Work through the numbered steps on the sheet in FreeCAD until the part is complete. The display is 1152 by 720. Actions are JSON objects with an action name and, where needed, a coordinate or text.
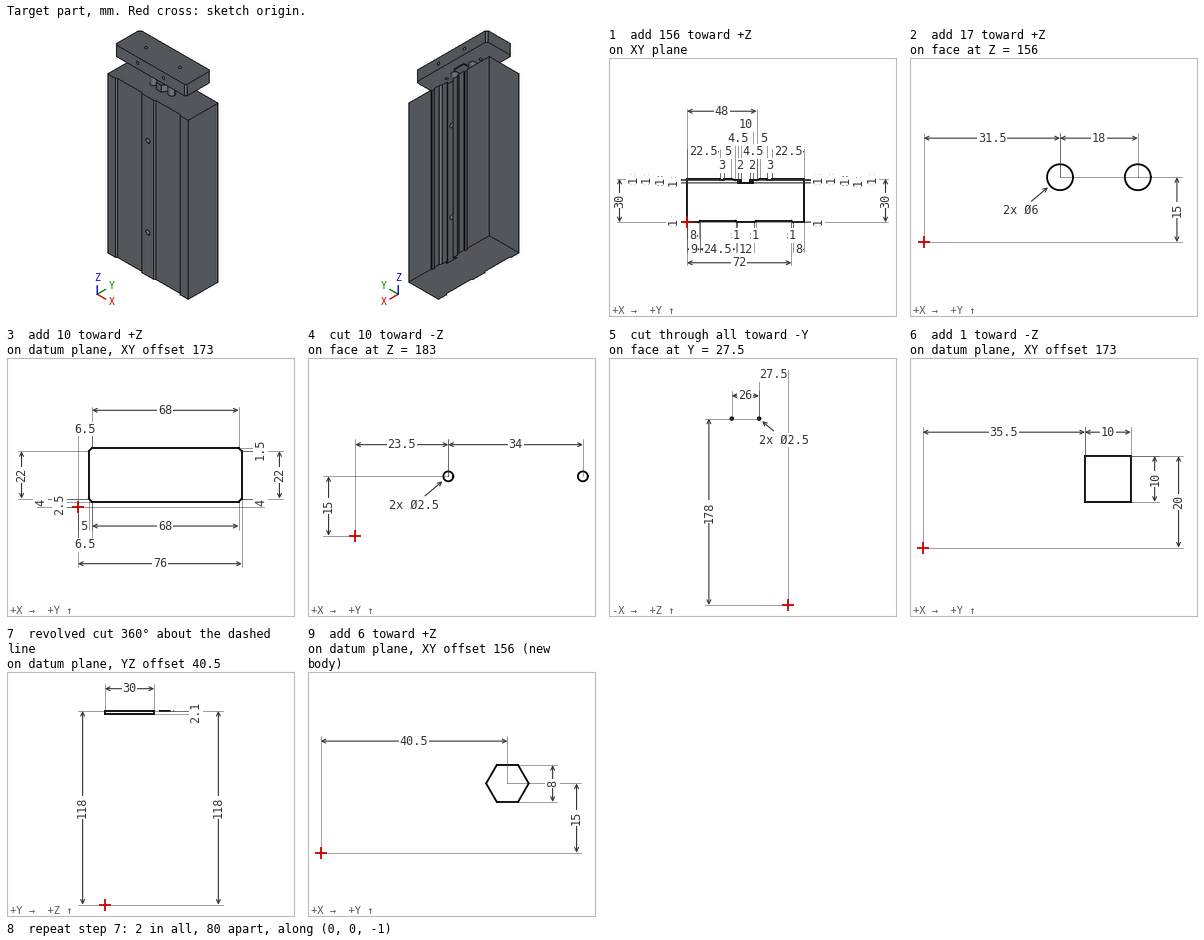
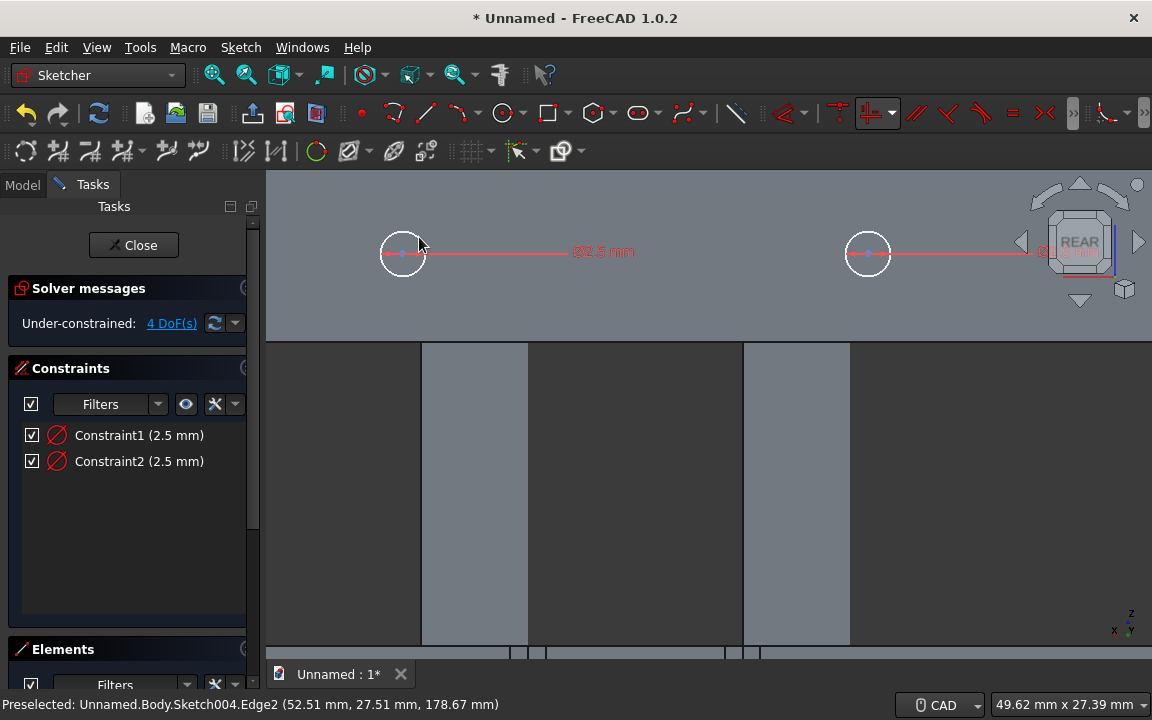
{"action": "left_click", "coordinate": [868, 254]}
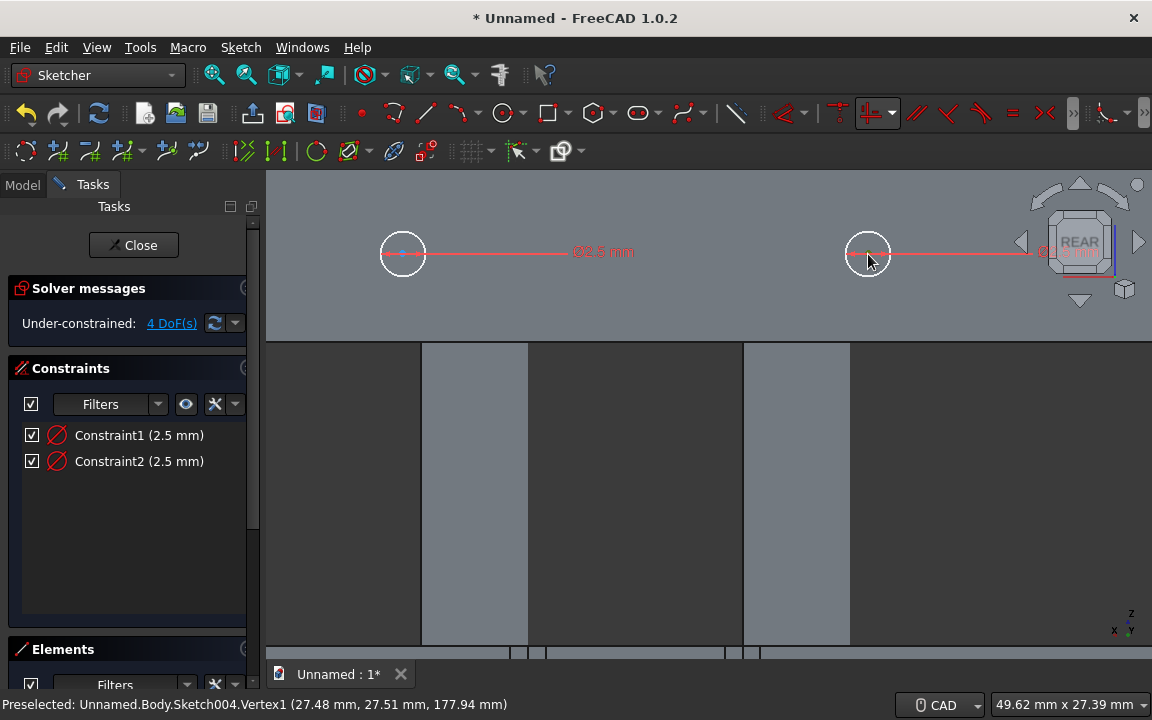
{"action": "left_click", "coordinate": [403, 254]}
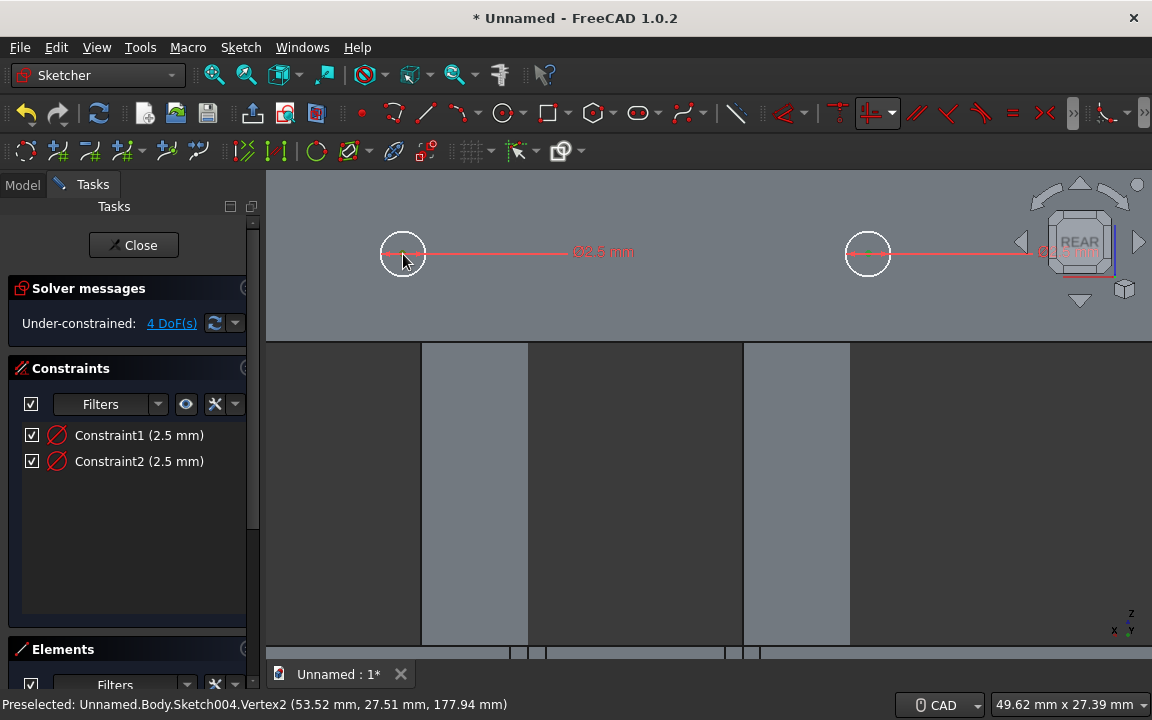
{"action": "key", "text": "h"}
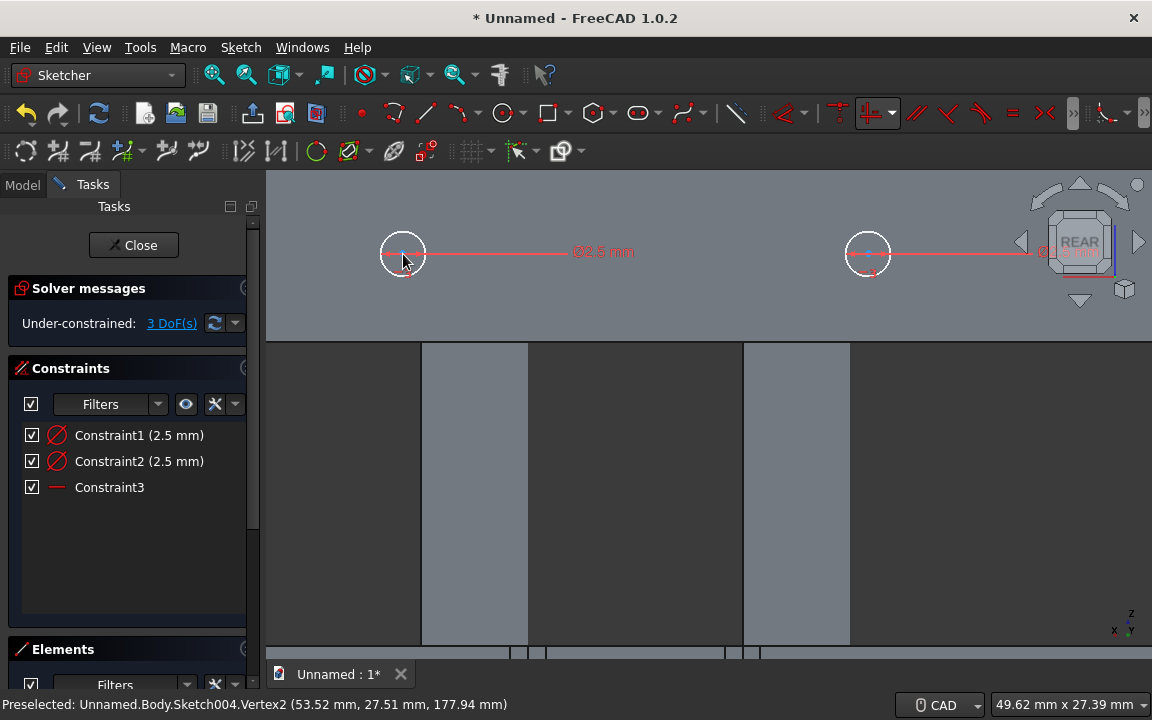
{"action": "key", "text": "d"}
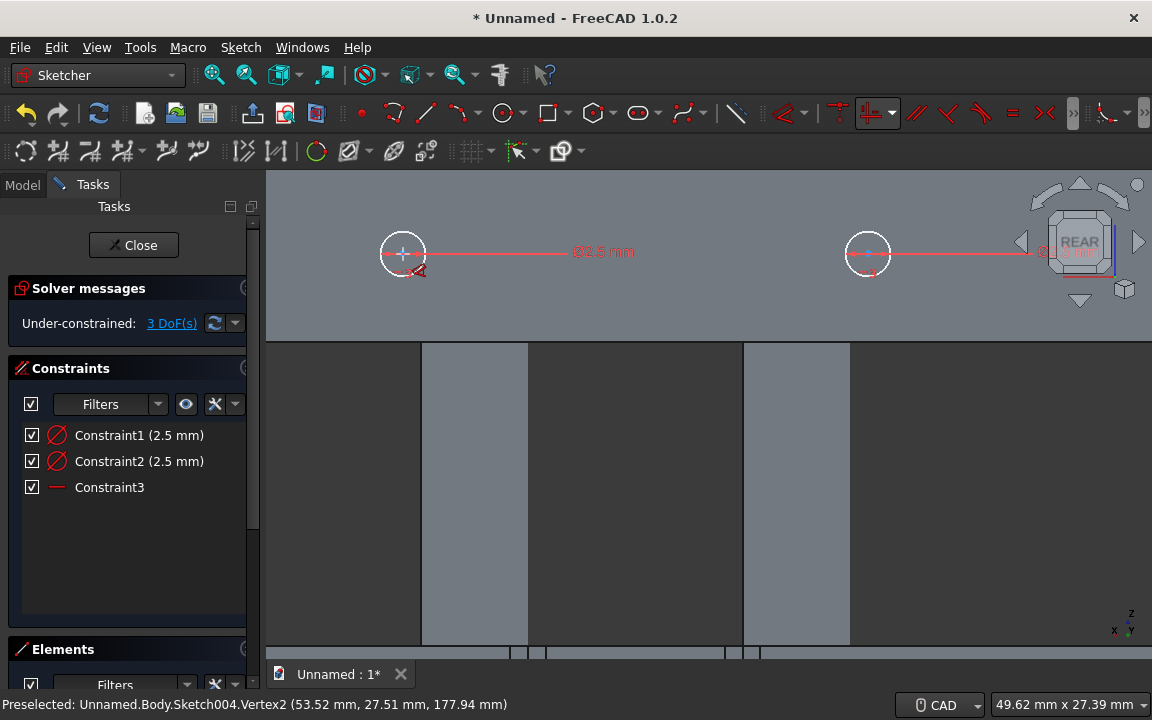
{"action": "left_click", "coordinate": [868, 254]}
{"action": "left_click", "coordinate": [834, 443]}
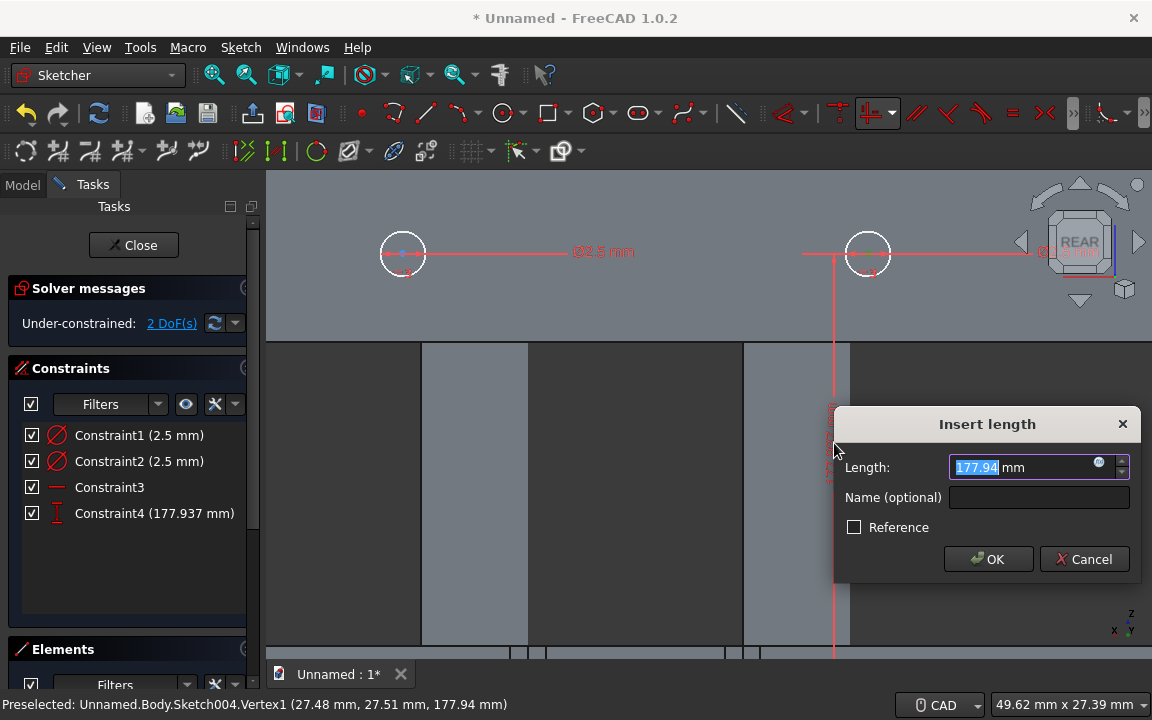
{"action": "type", "text": "178"}
{"action": "key", "text": "Return"}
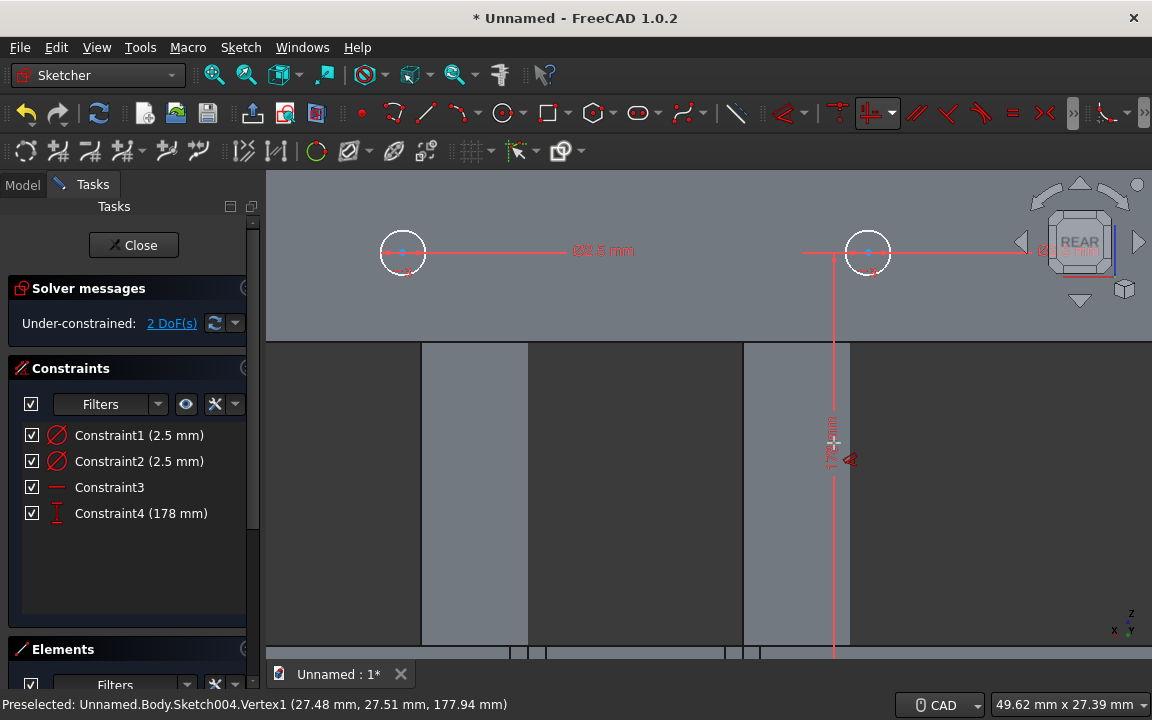
{"action": "left_click", "coordinate": [868, 253]}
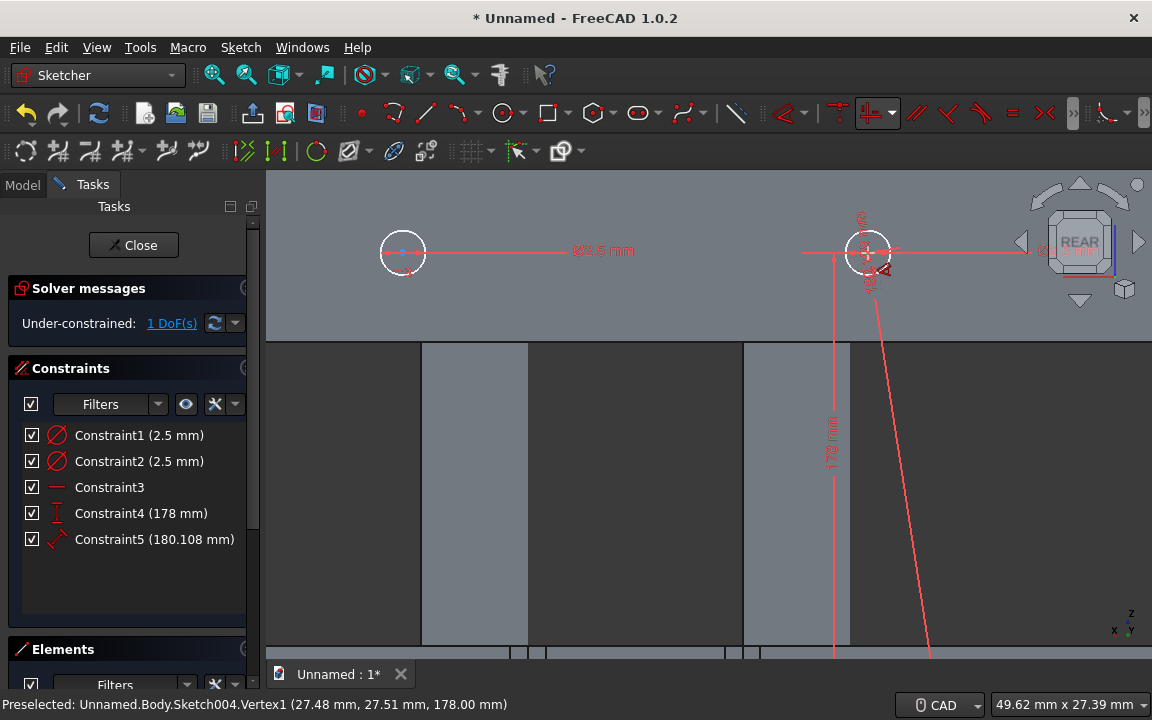
{"action": "left_click", "coordinate": [403, 253]}
{"action": "left_click", "coordinate": [636, 287]}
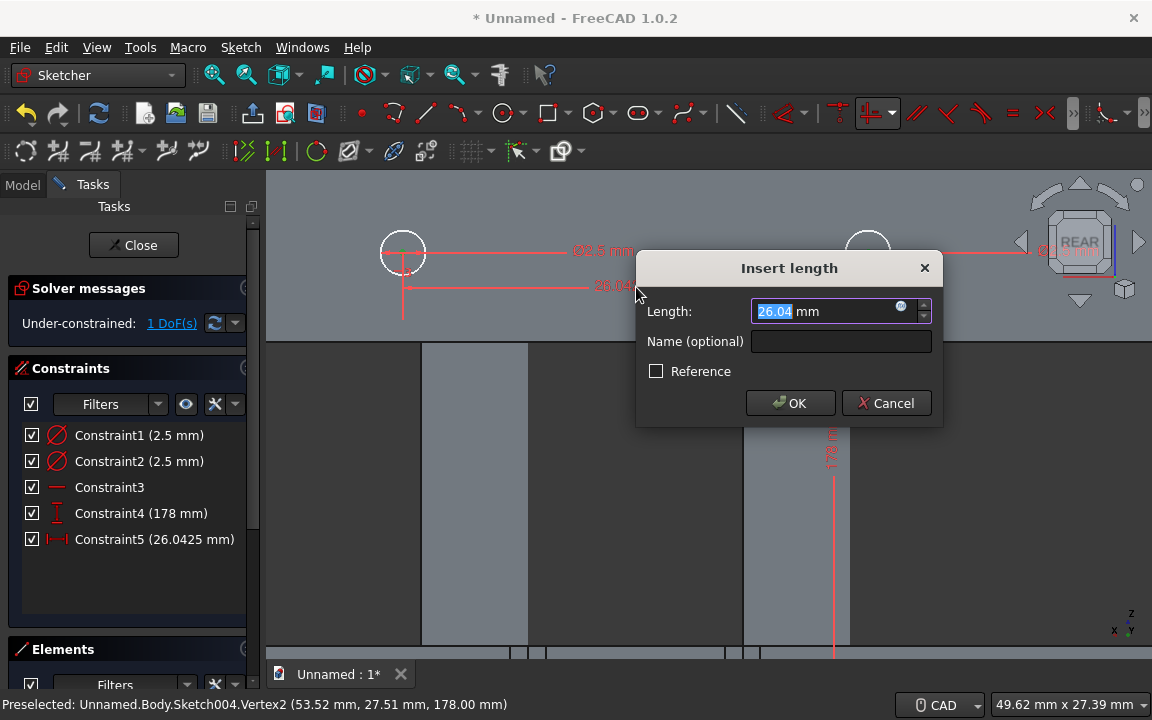
{"action": "type", "text": "26"}
{"action": "key", "text": "Return"}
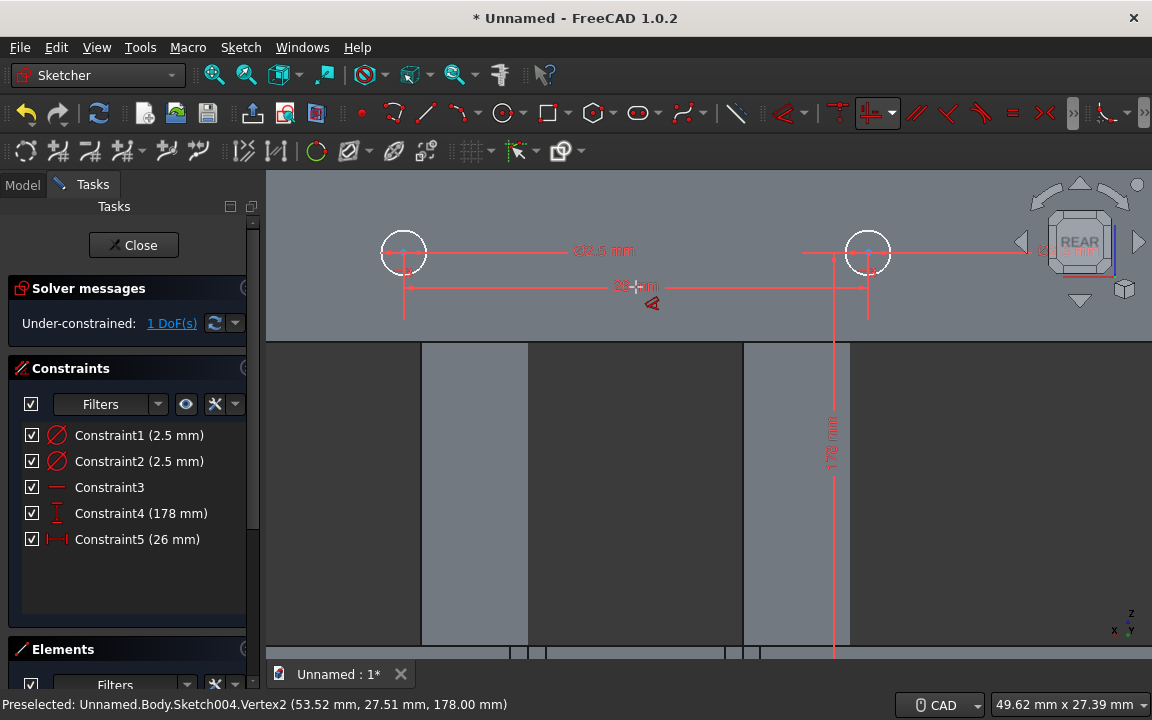
{"action": "left_click", "coordinate": [868, 253]}
{"action": "left_click", "coordinate": [928, 219]}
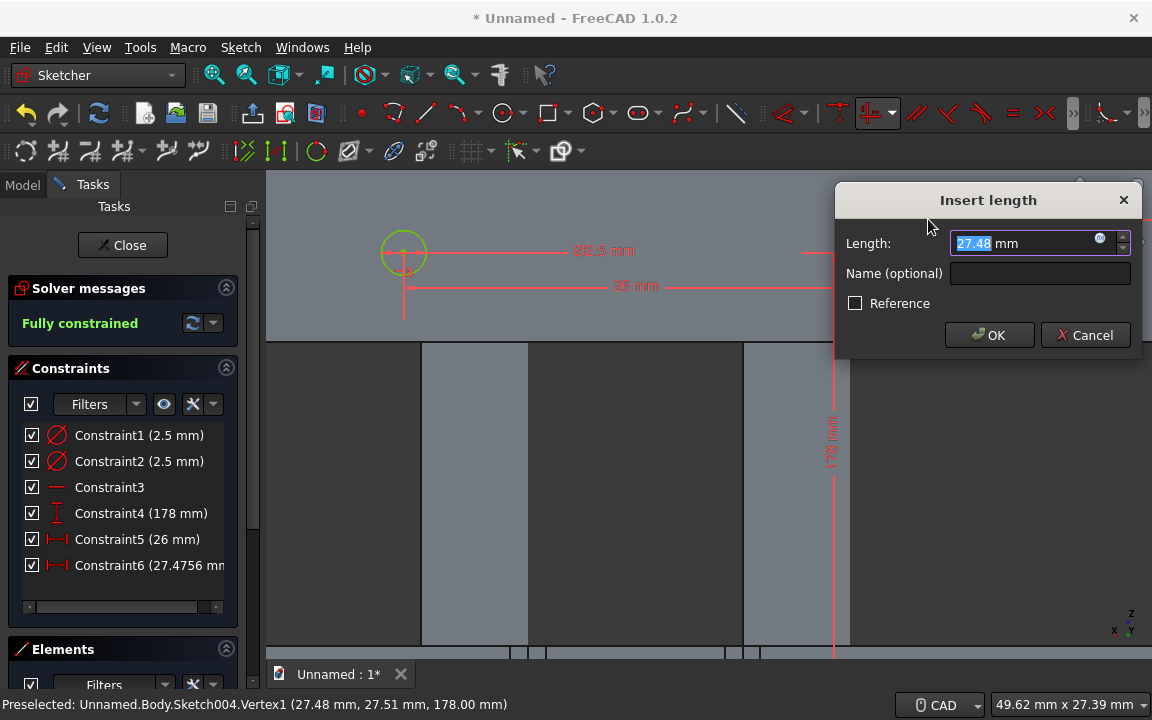
{"action": "type", "text": "27.5"}
{"action": "key", "text": "Return"}
{"action": "key", "text": "Escape"}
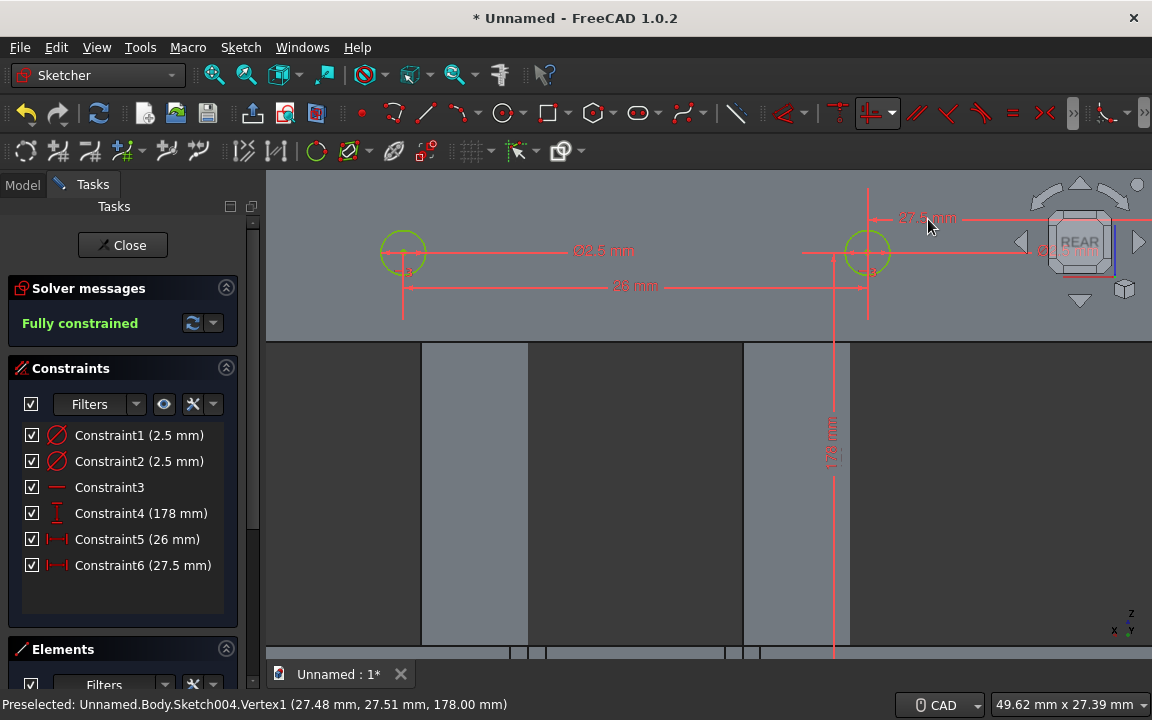
{"action": "left_click", "coordinate": [123, 245]}